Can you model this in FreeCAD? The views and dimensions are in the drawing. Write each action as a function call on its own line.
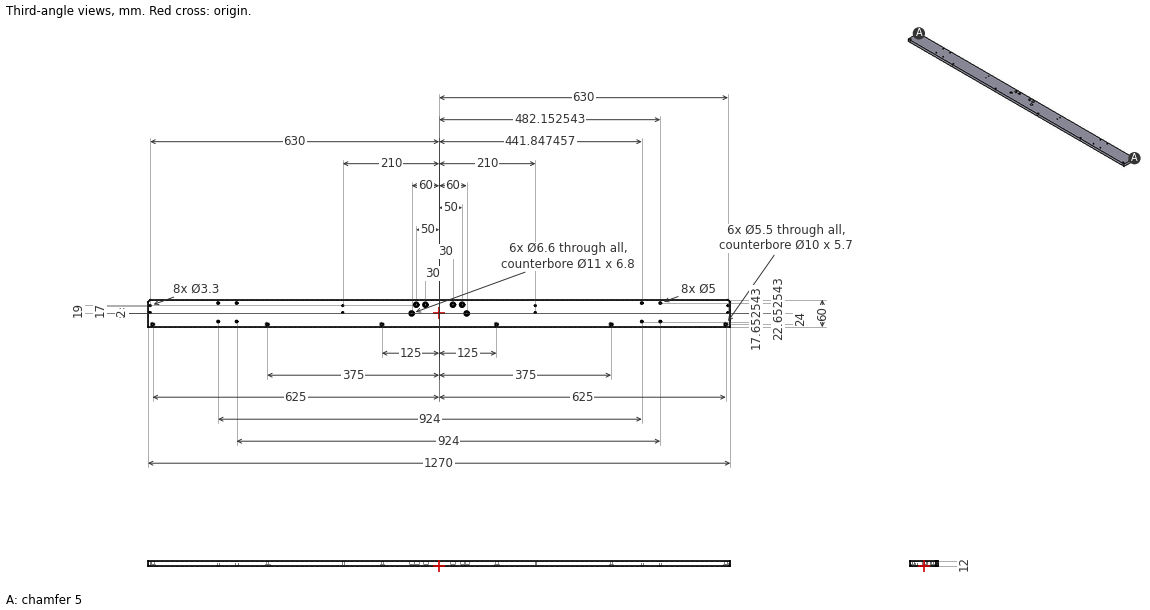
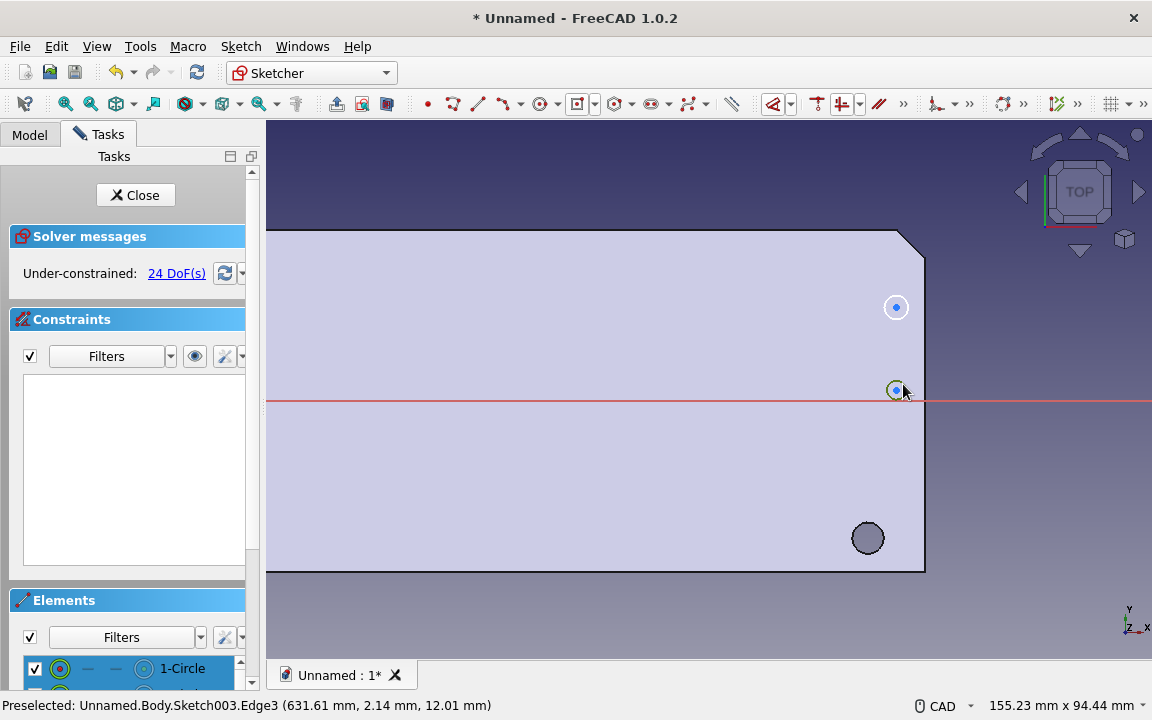
click(905, 299)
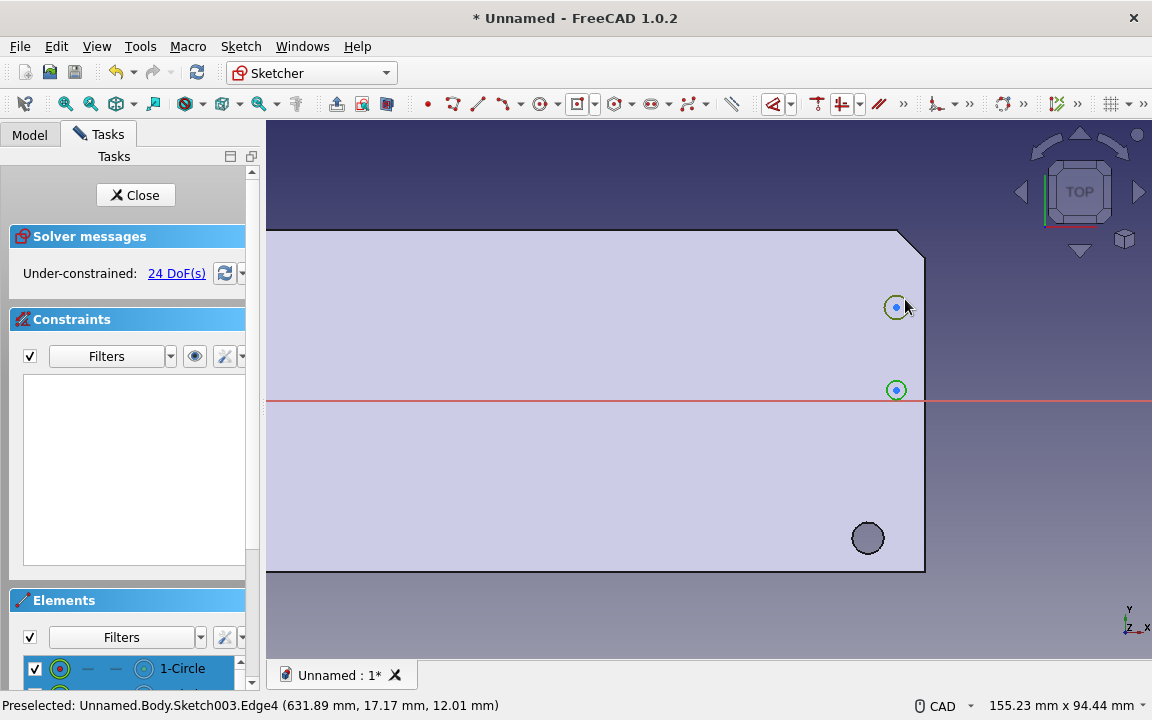
scroll(908, 393, down, 13)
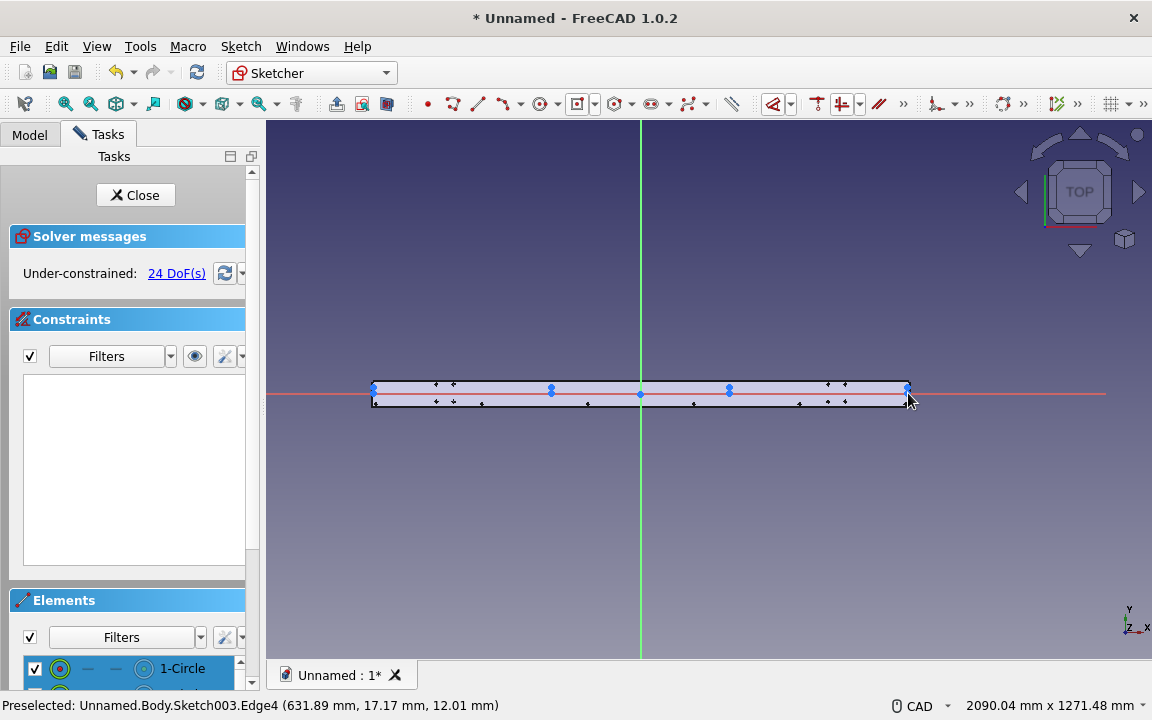
scroll(552, 387, up, 13)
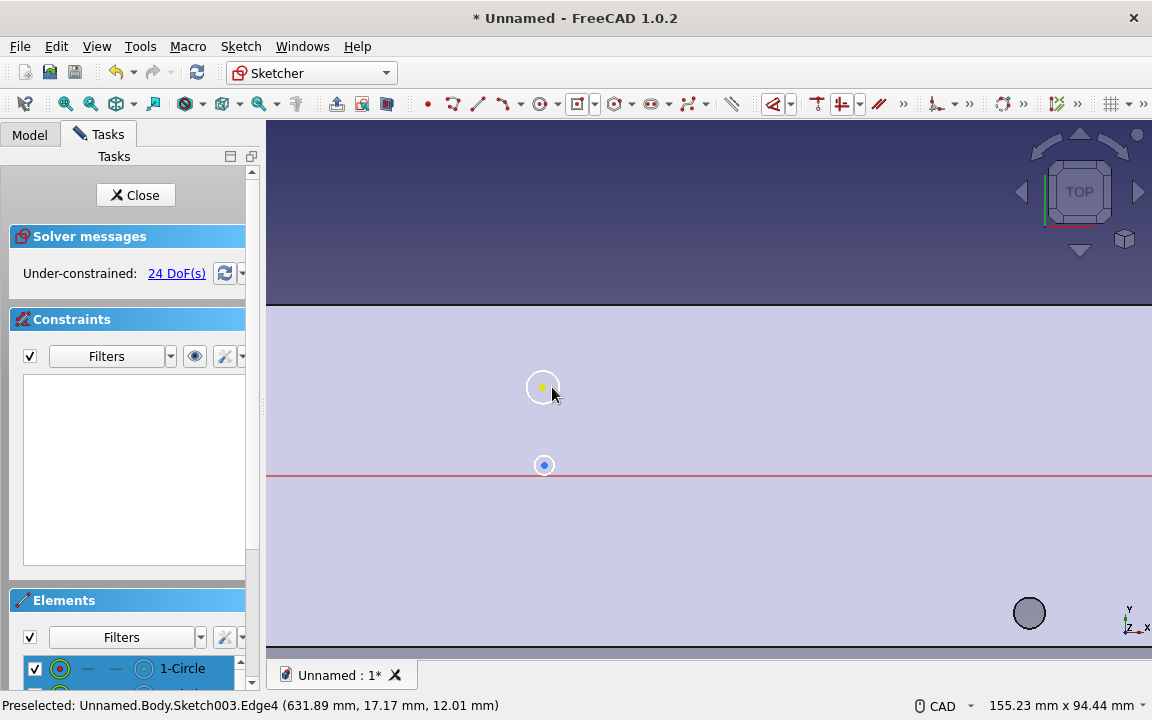
click(554, 376)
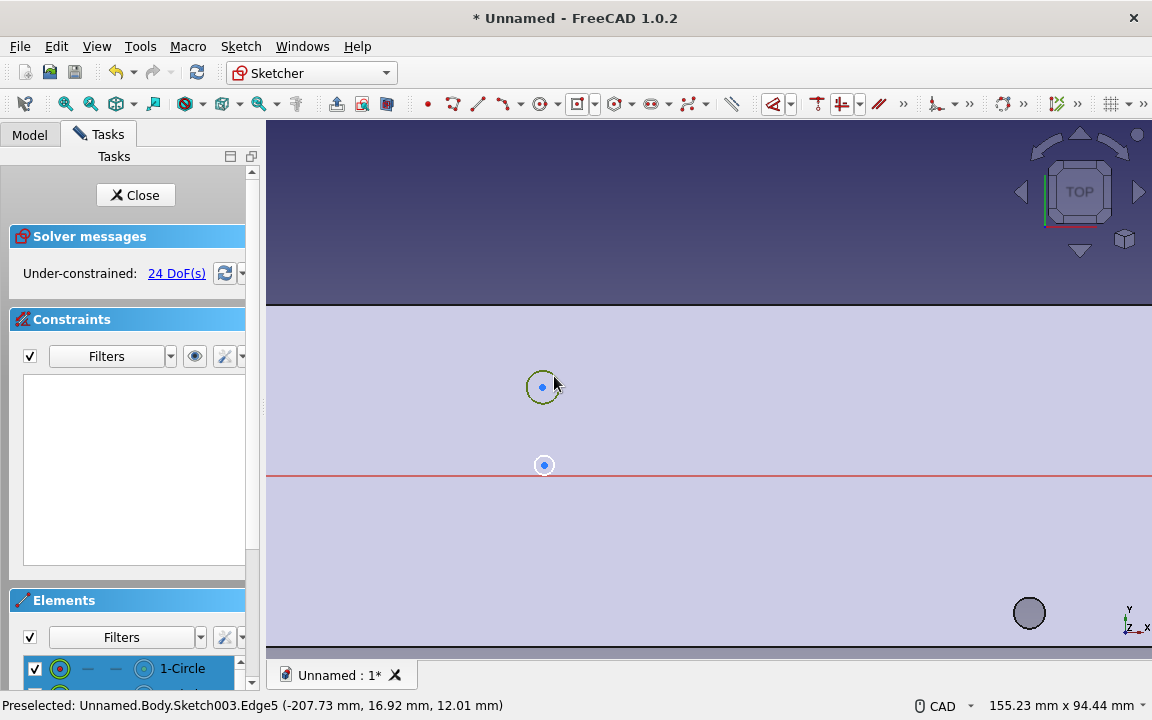
click(551, 458)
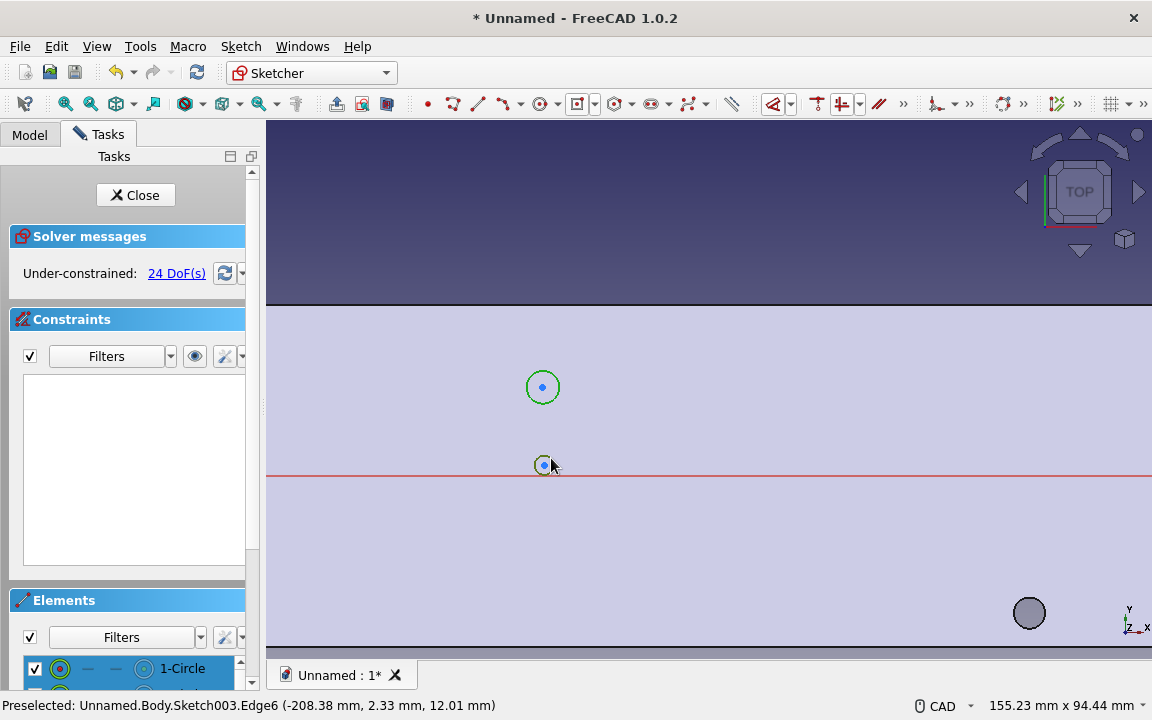
scroll(552, 387, down, 13)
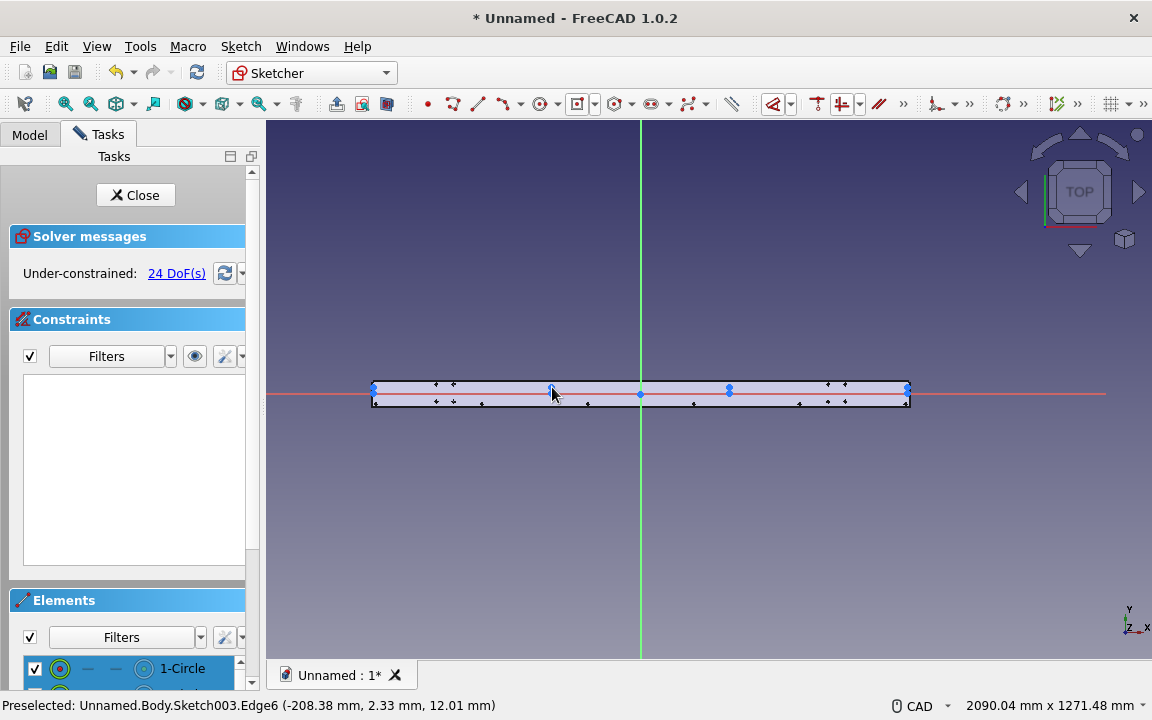
scroll(730, 393, up, 13)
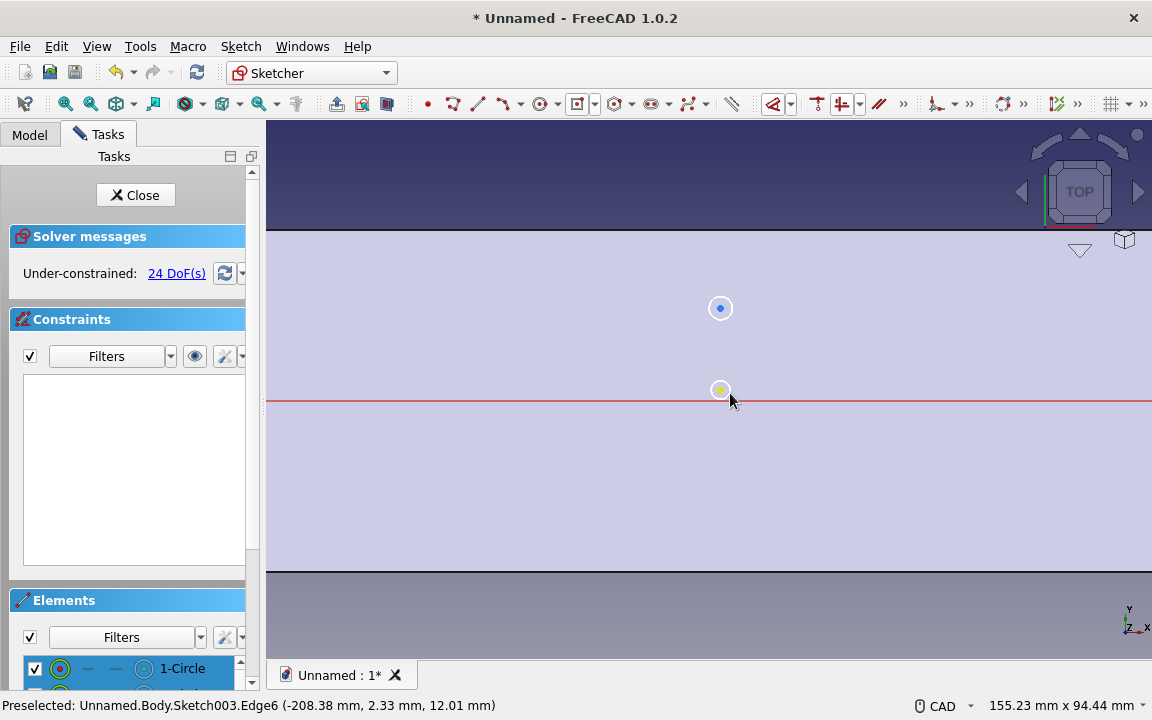
click(727, 383)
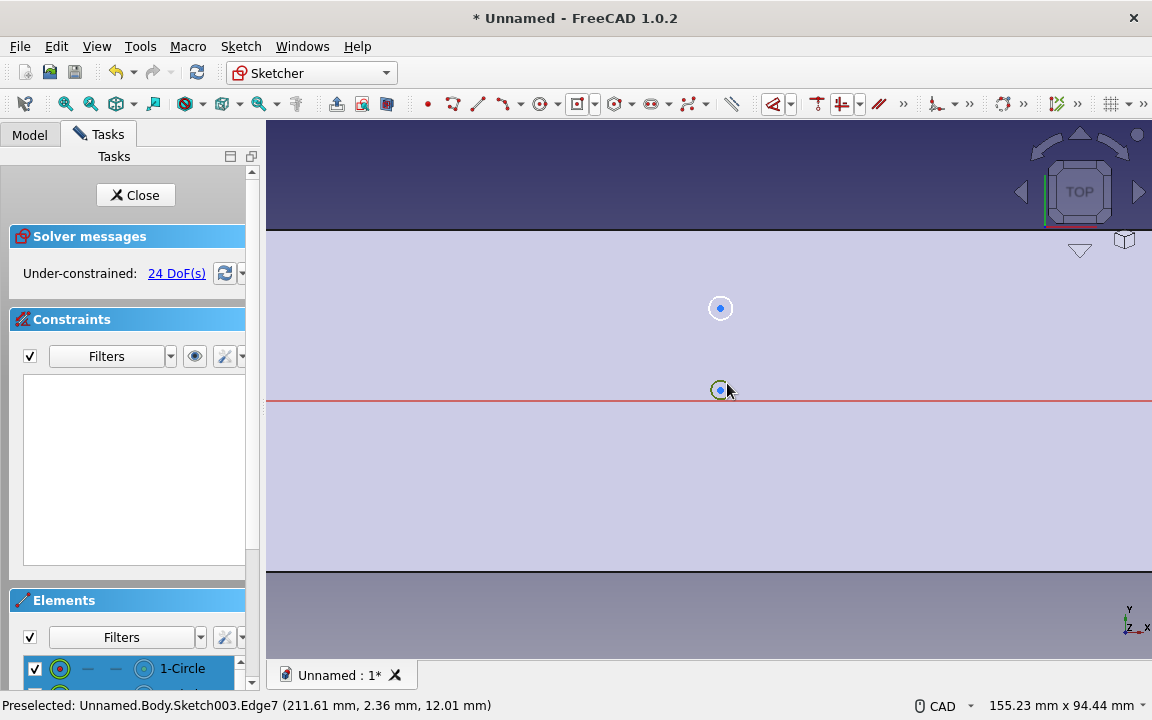
click(729, 300)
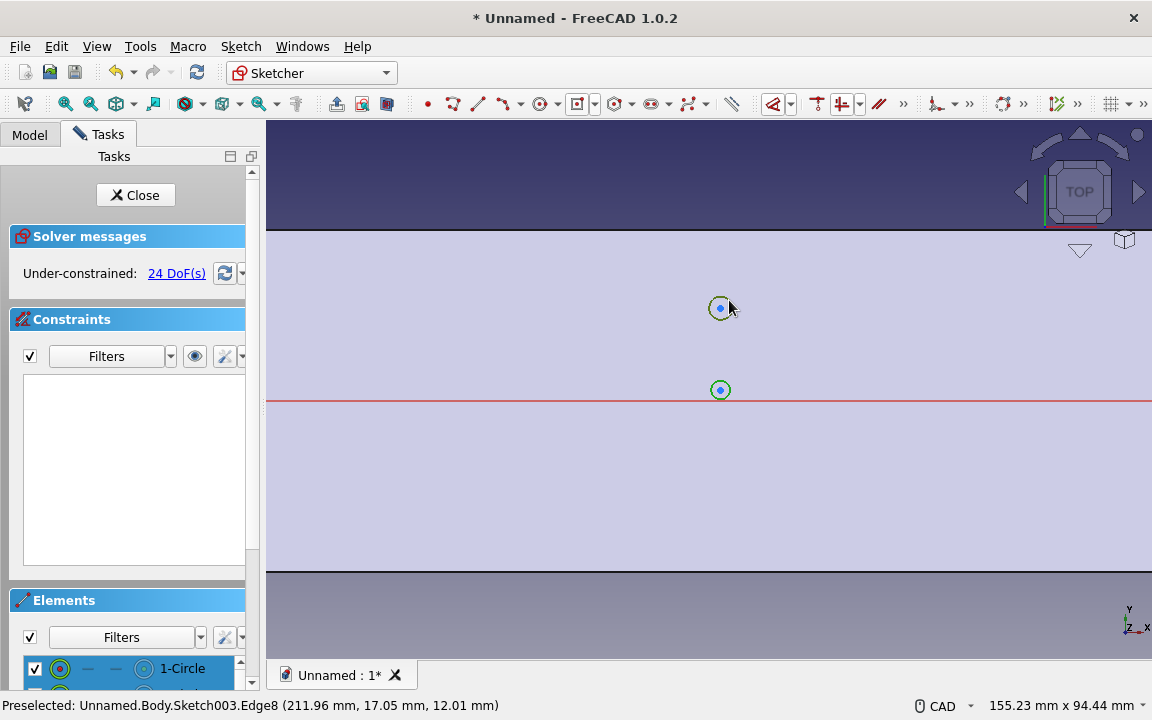
key(e)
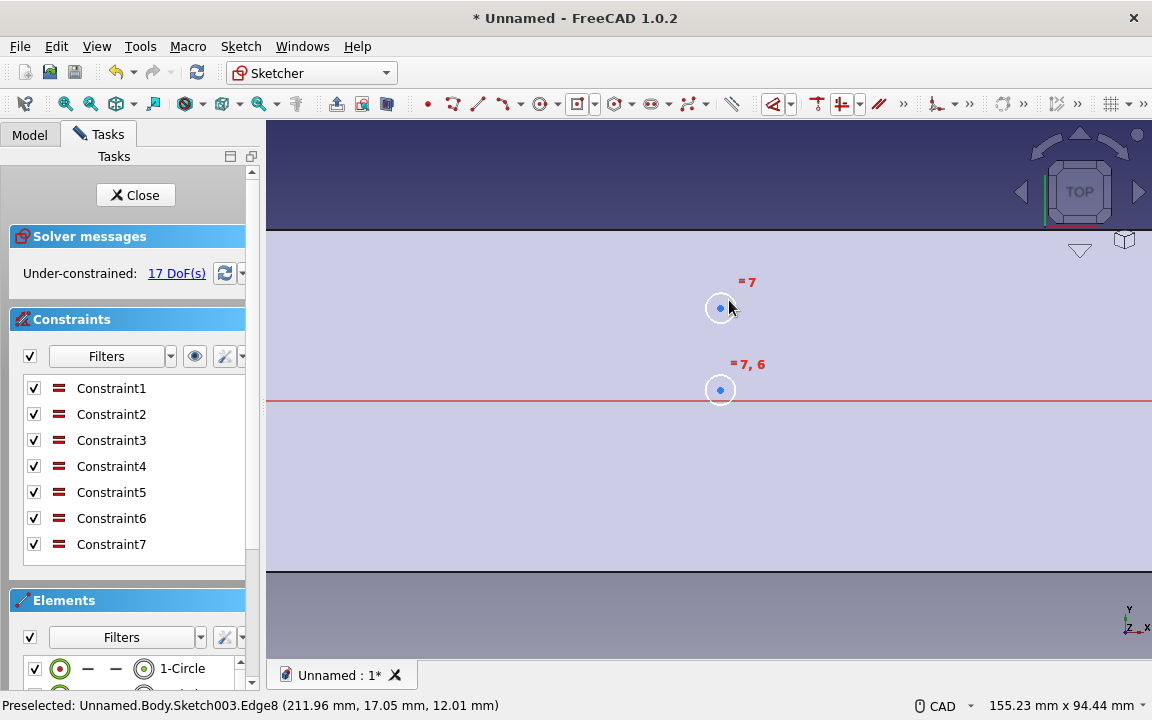
scroll(730, 393, down, 13)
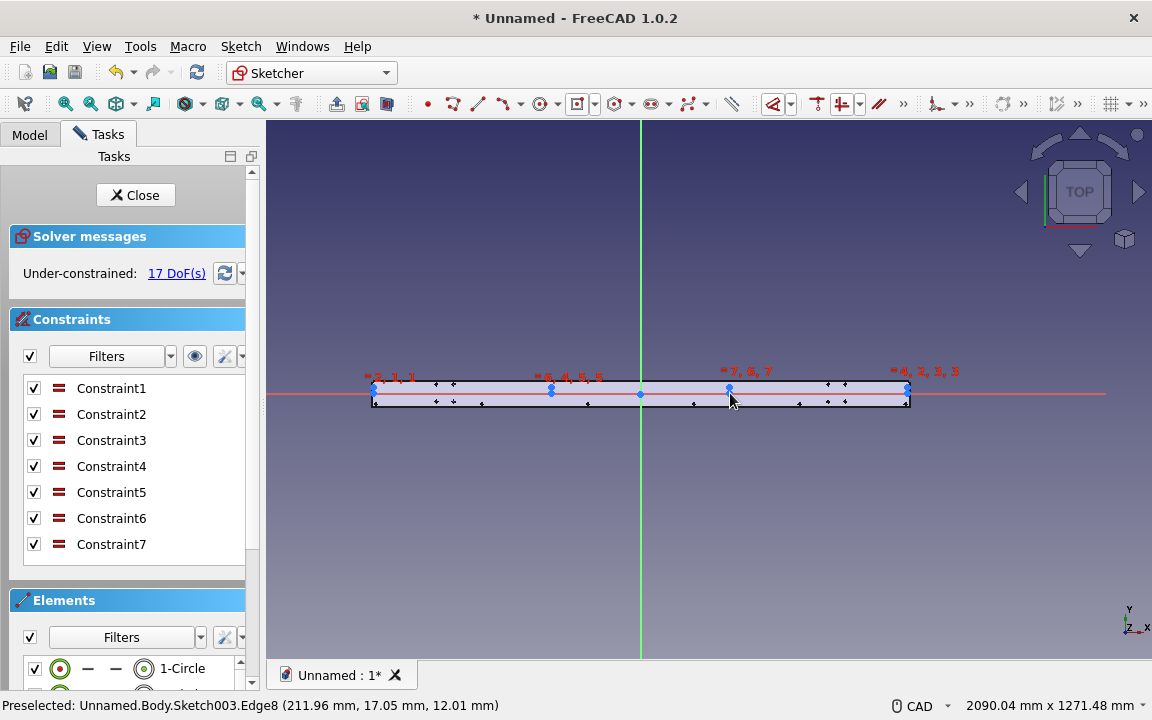
scroll(374, 387, up, 4)